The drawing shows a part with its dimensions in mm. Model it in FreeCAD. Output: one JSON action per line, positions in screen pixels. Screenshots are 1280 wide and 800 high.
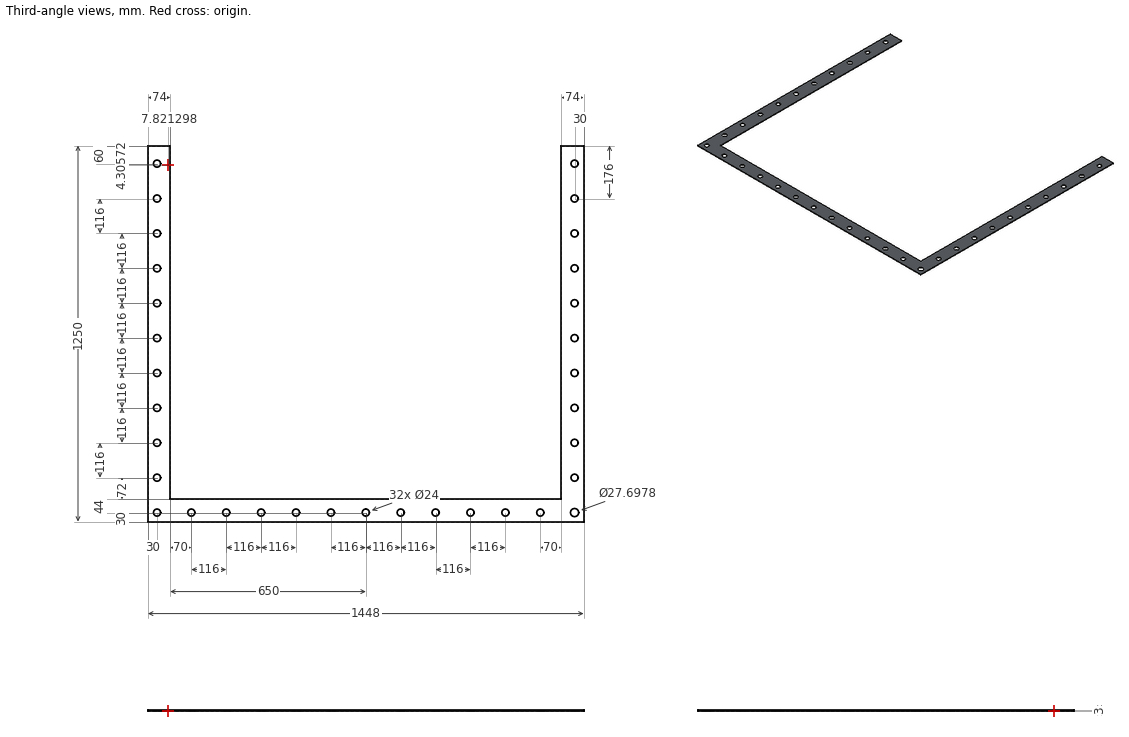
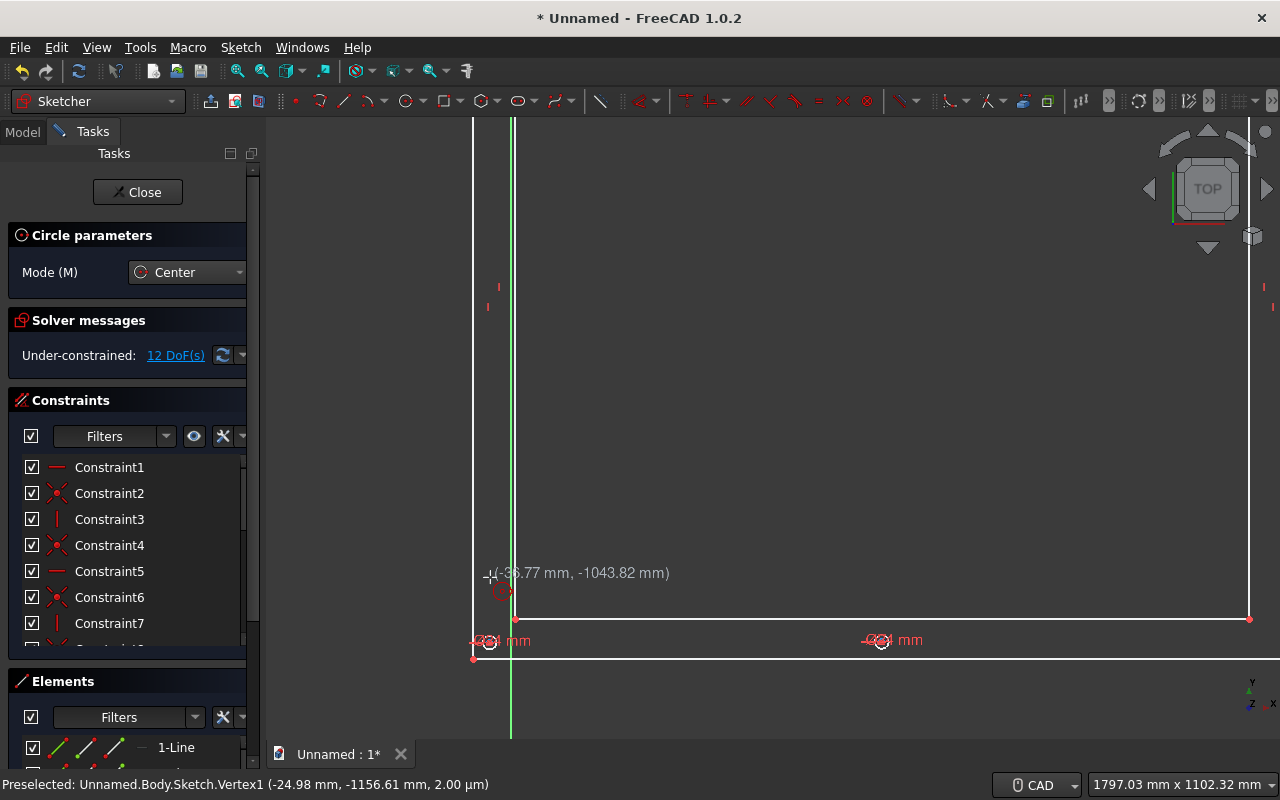
{"action": "left_click", "coordinate": [490, 576]}
{"action": "mouse_move", "coordinate": [495, 571]}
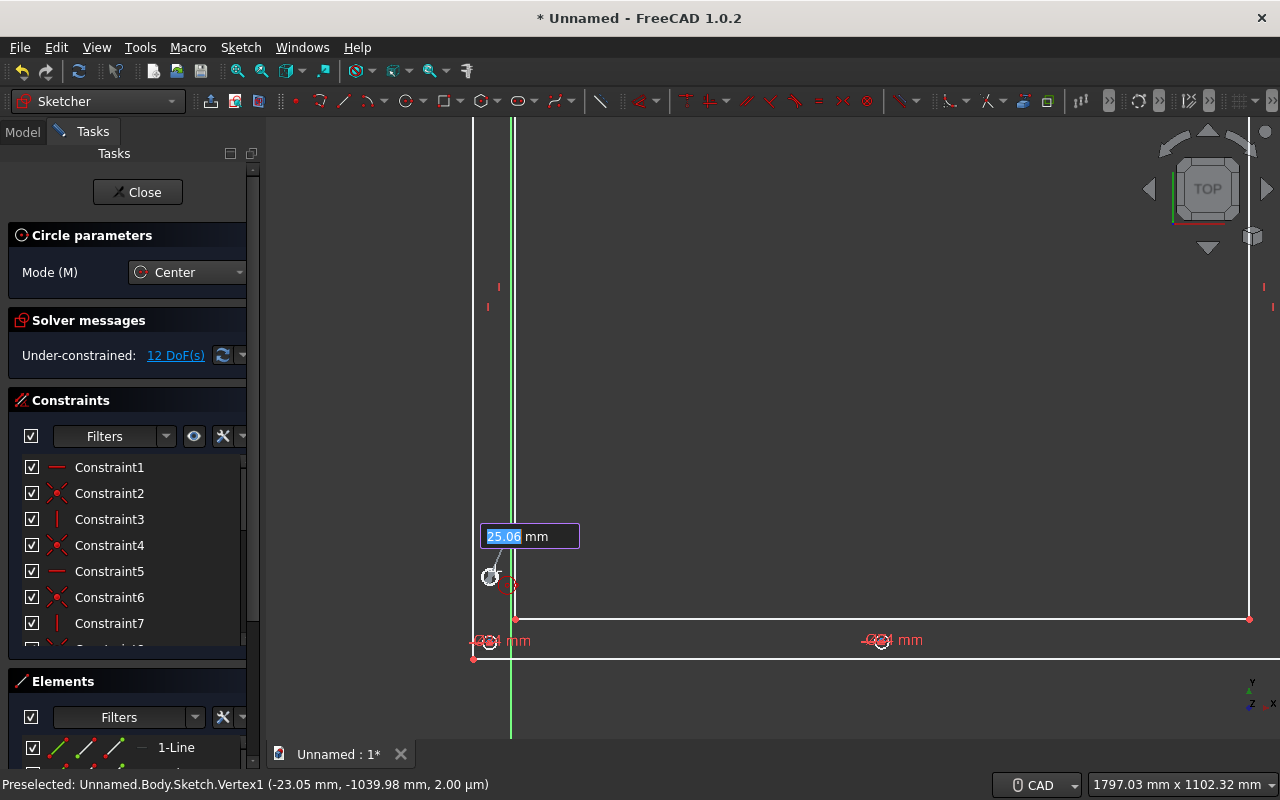
{"action": "type", "text": "24"}
{"action": "key", "text": "Return"}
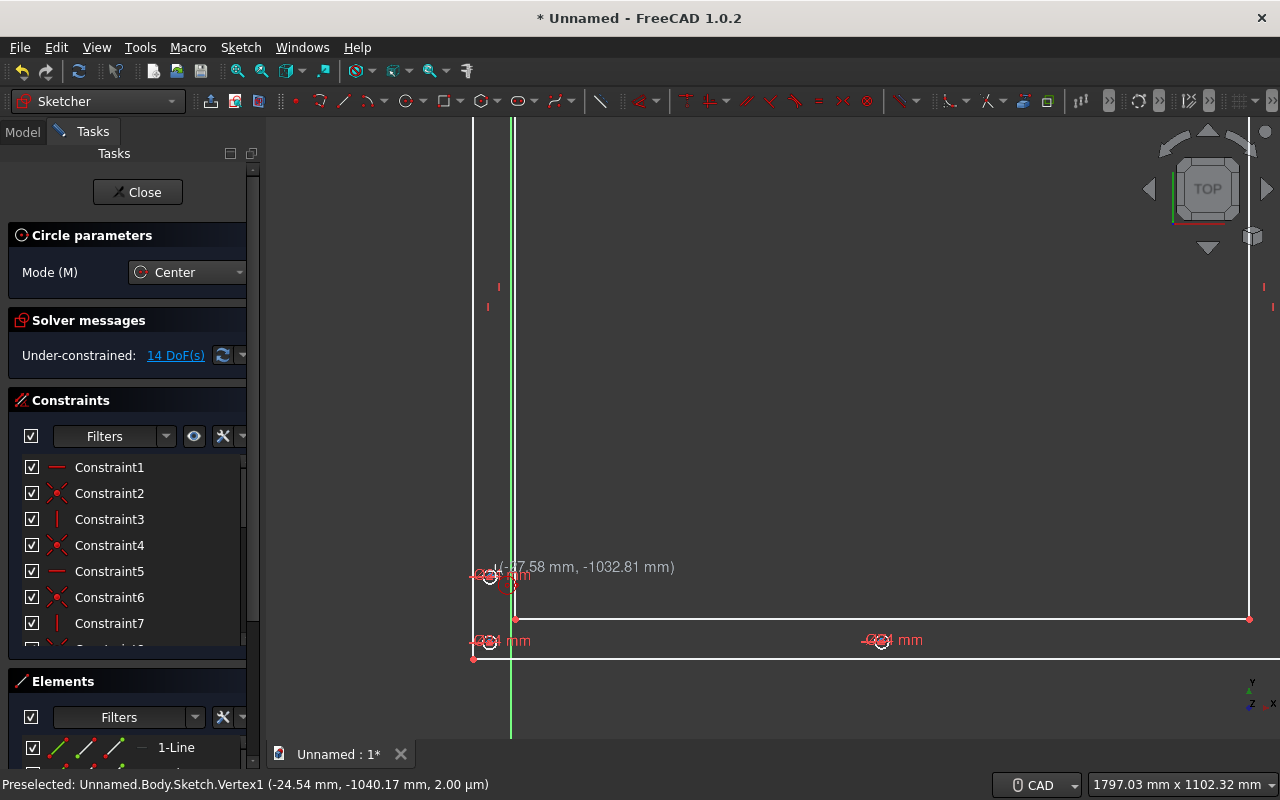
{"action": "scroll", "coordinate": [554, 641], "scroll_direction": "up", "scroll_amount": 7}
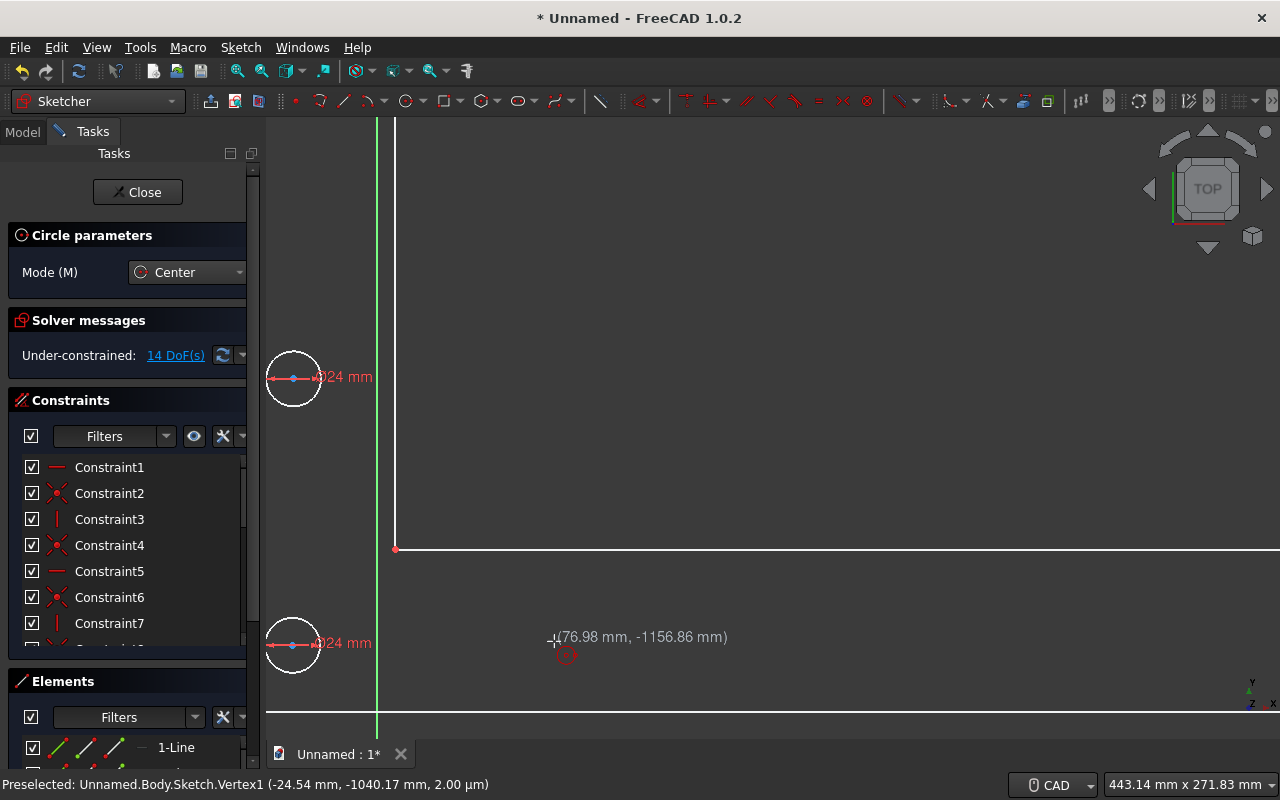
{"action": "scroll", "coordinate": [520, 608], "scroll_direction": "down", "scroll_amount": 10}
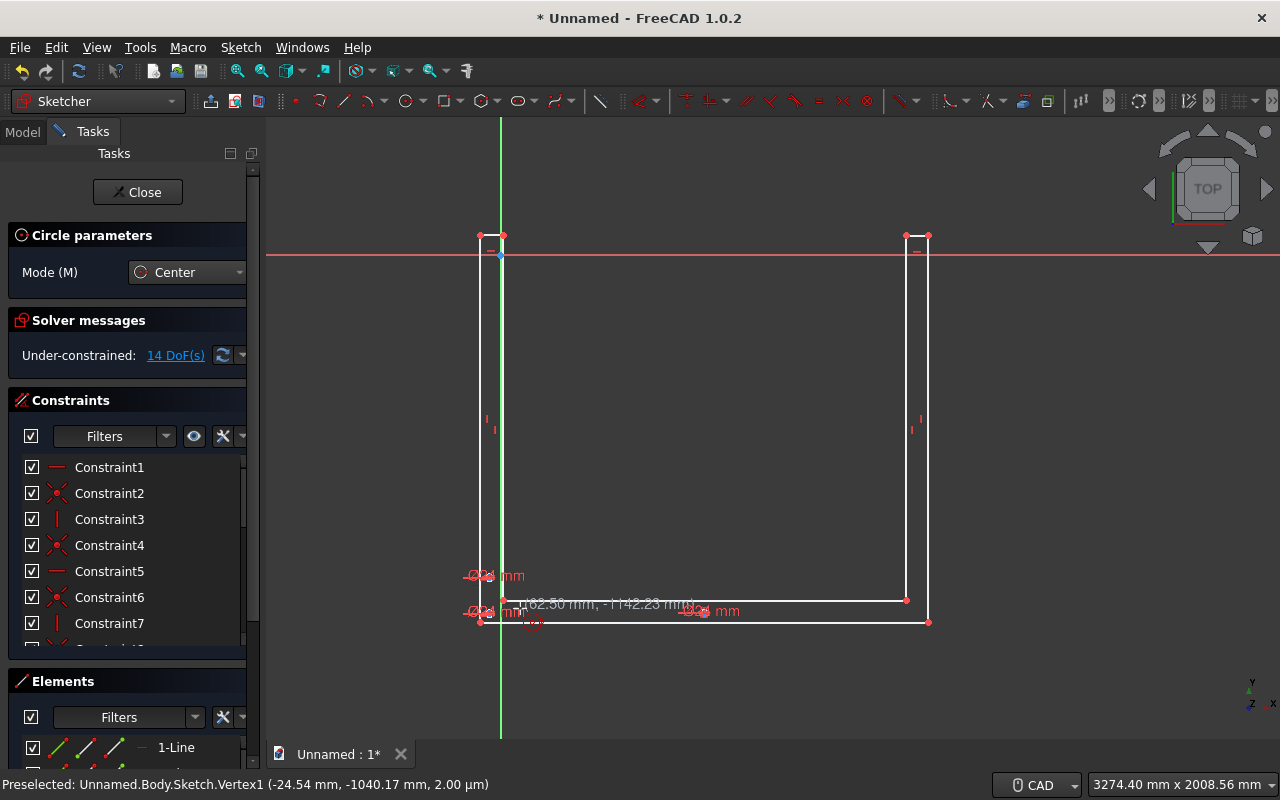
{"action": "scroll", "coordinate": [525, 613], "scroll_direction": "up", "scroll_amount": 3}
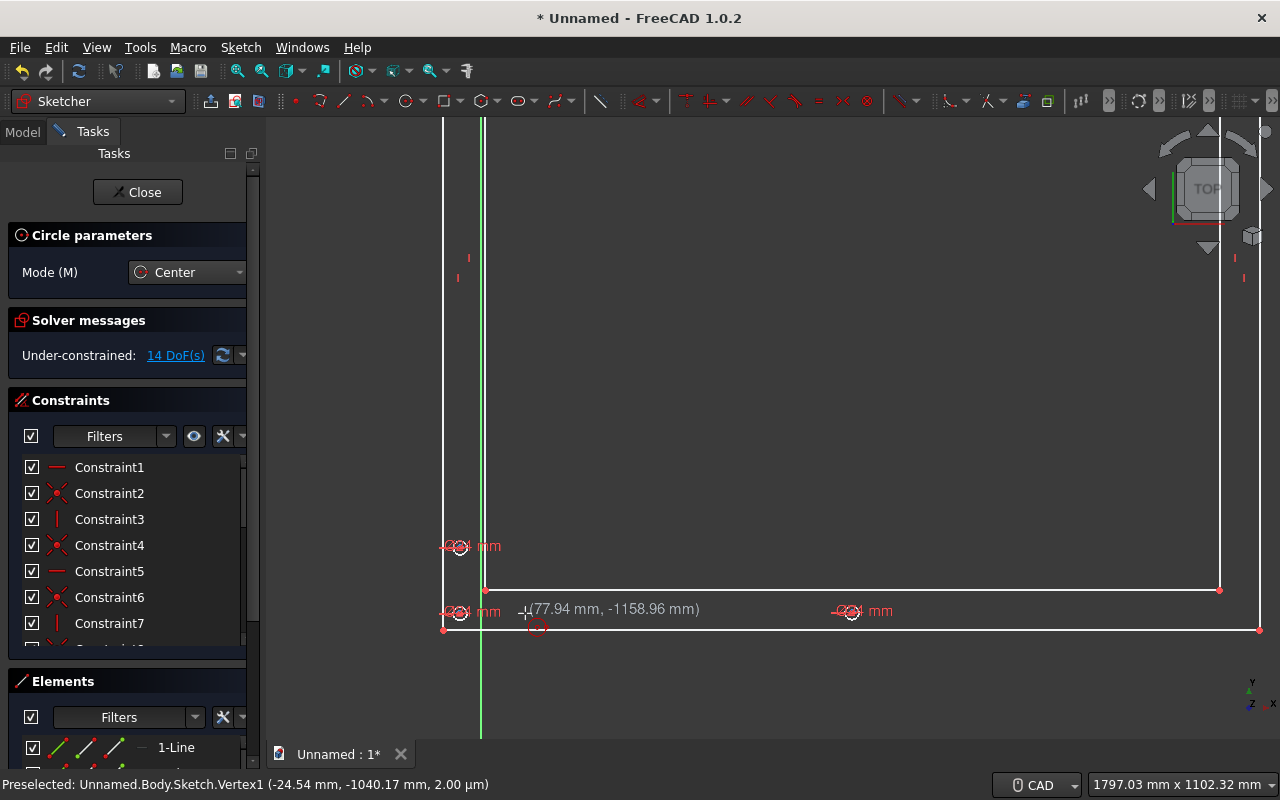
{"action": "left_click", "coordinate": [525, 612]}
{"action": "mouse_move", "coordinate": [530, 608]}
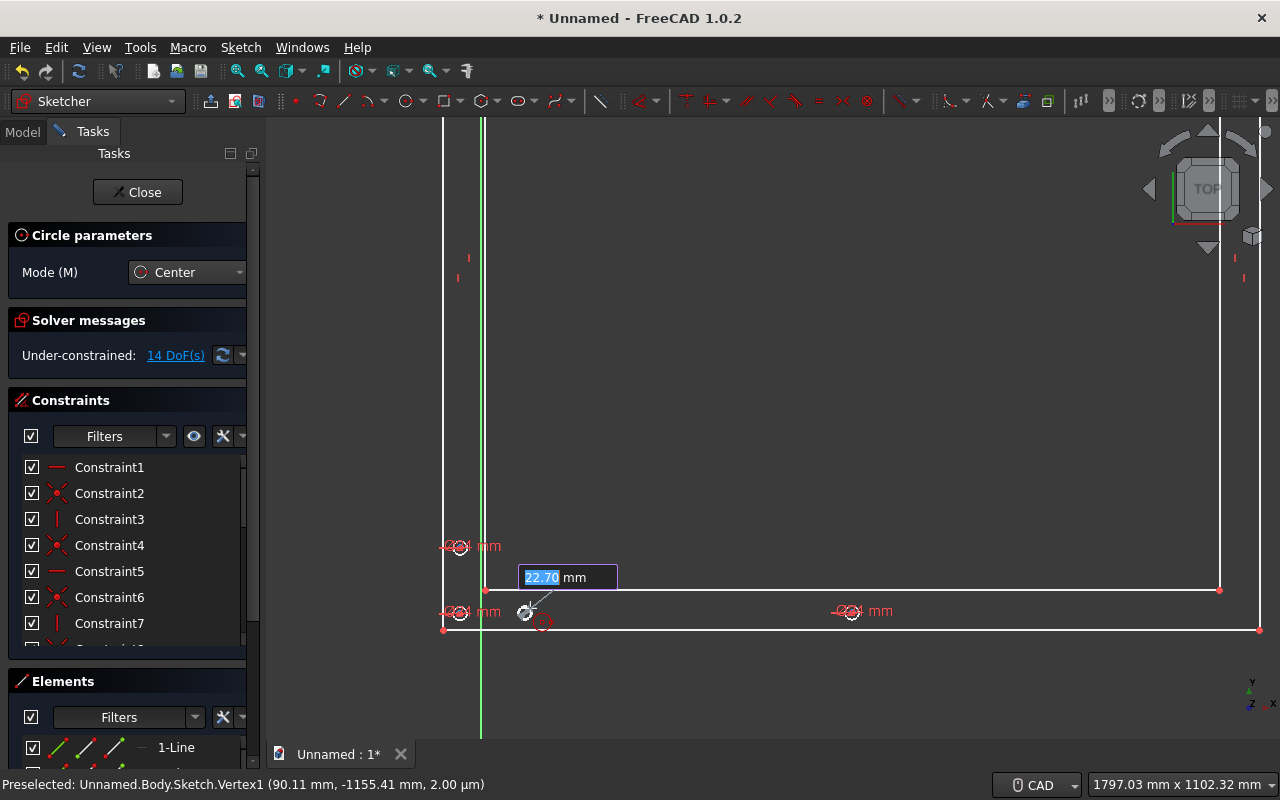
{"action": "type", "text": "24"}
{"action": "key", "text": "Return"}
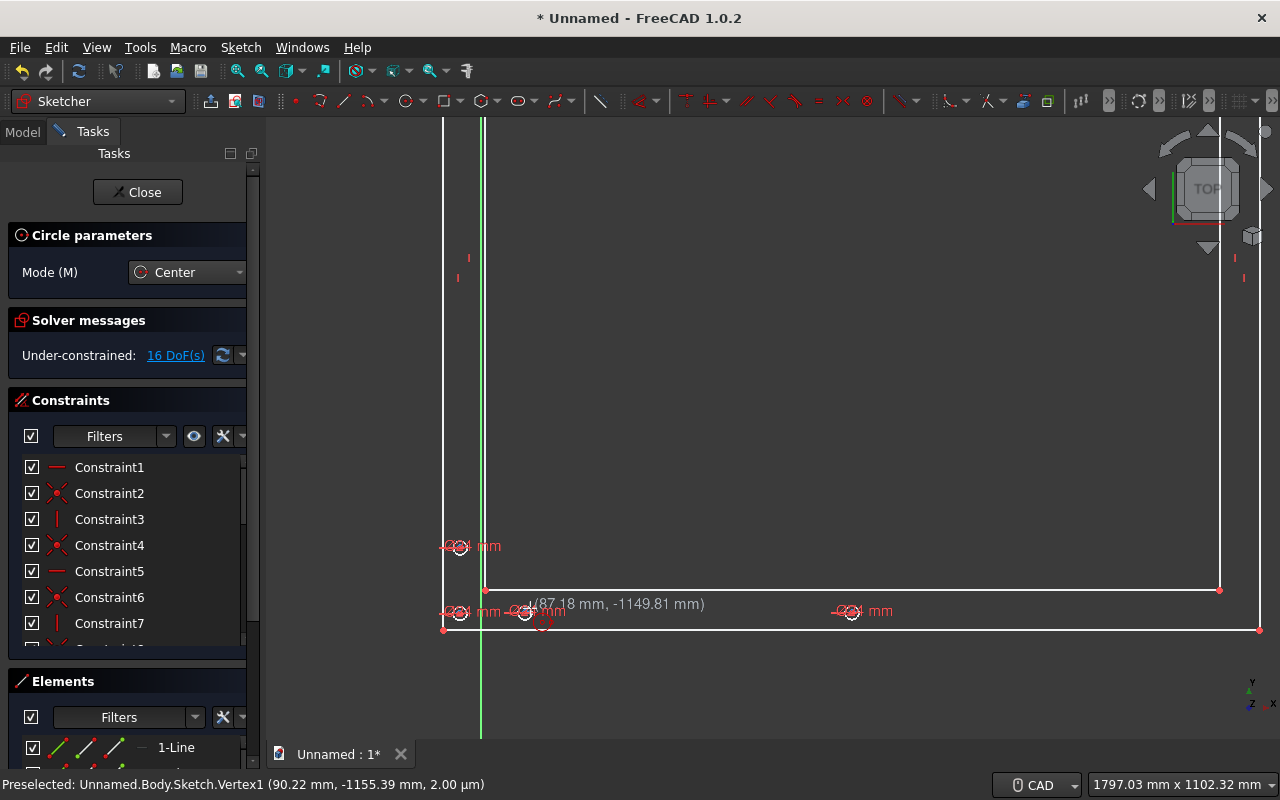
{"action": "scroll", "coordinate": [460, 481], "scroll_direction": "up", "scroll_amount": 7}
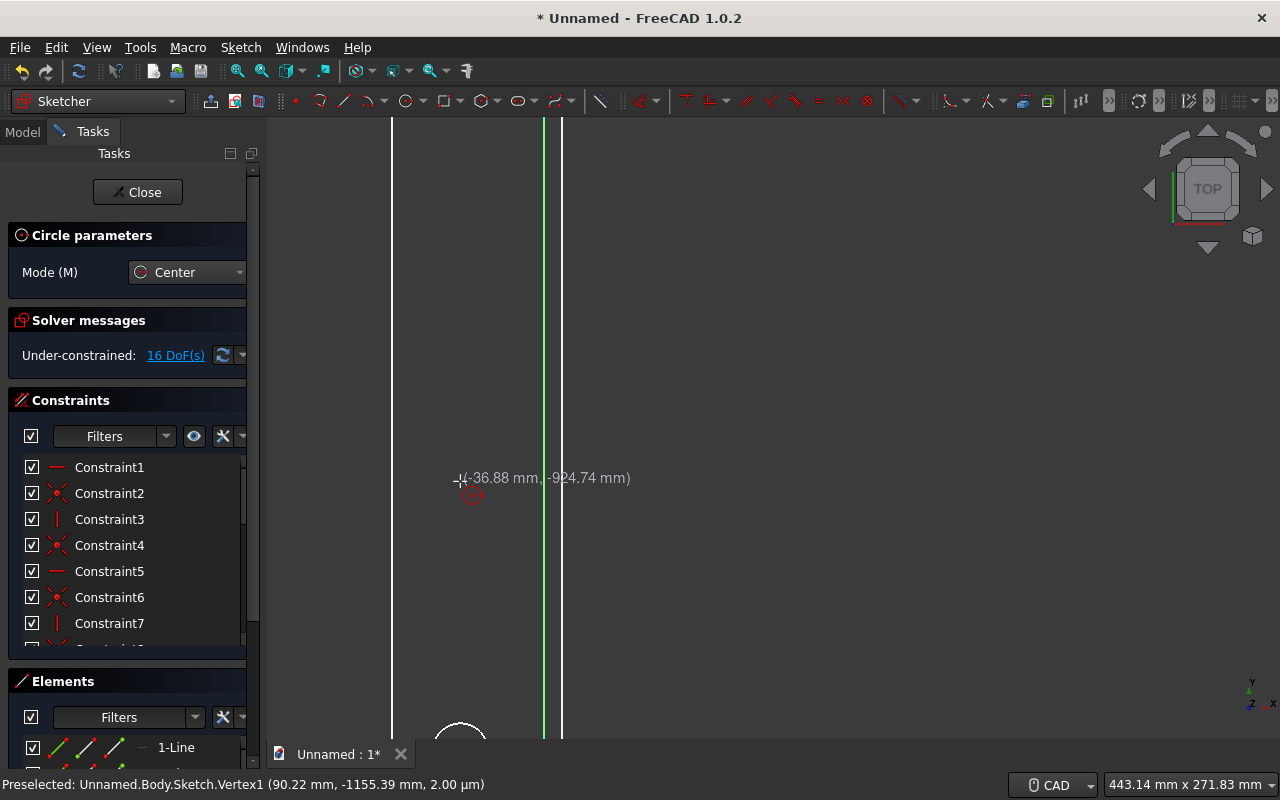
{"action": "scroll", "coordinate": [494, 550], "scroll_direction": "down", "scroll_amount": 10}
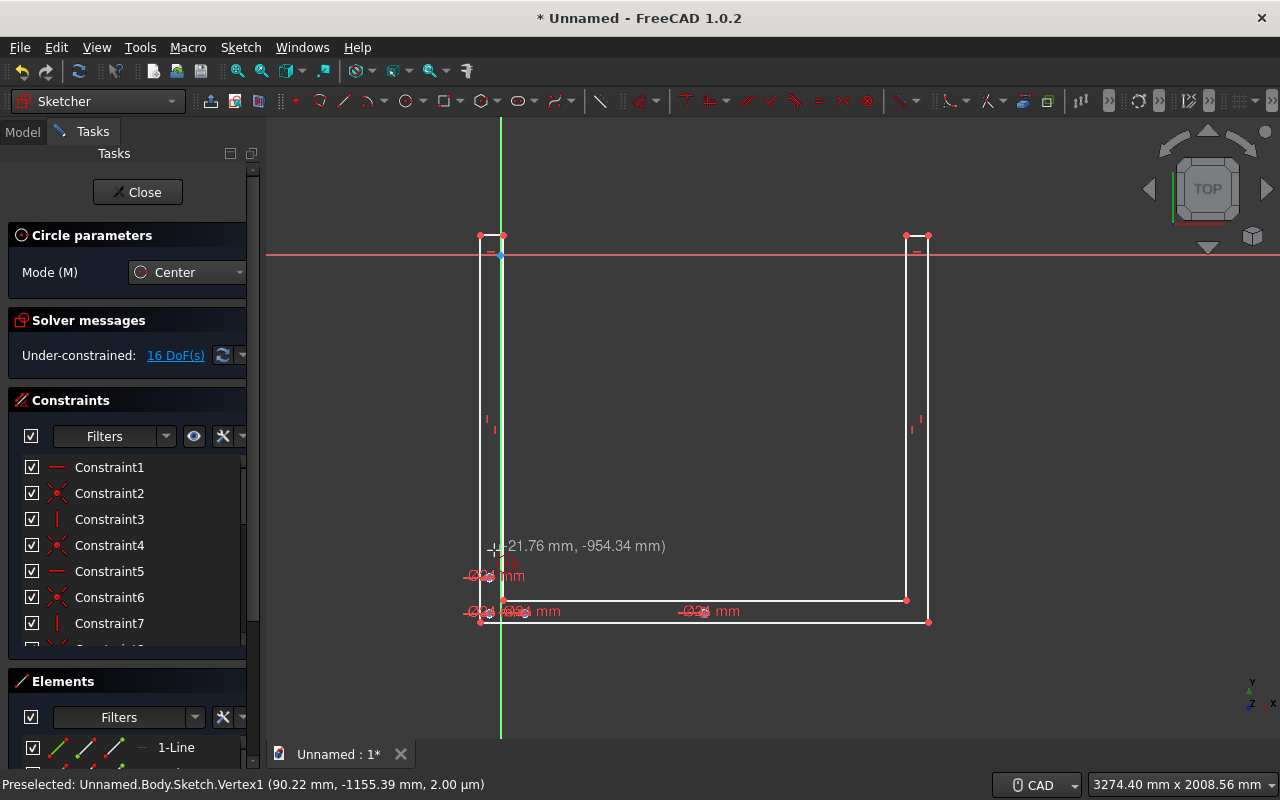
{"action": "scroll", "coordinate": [490, 541], "scroll_direction": "up", "scroll_amount": 3}